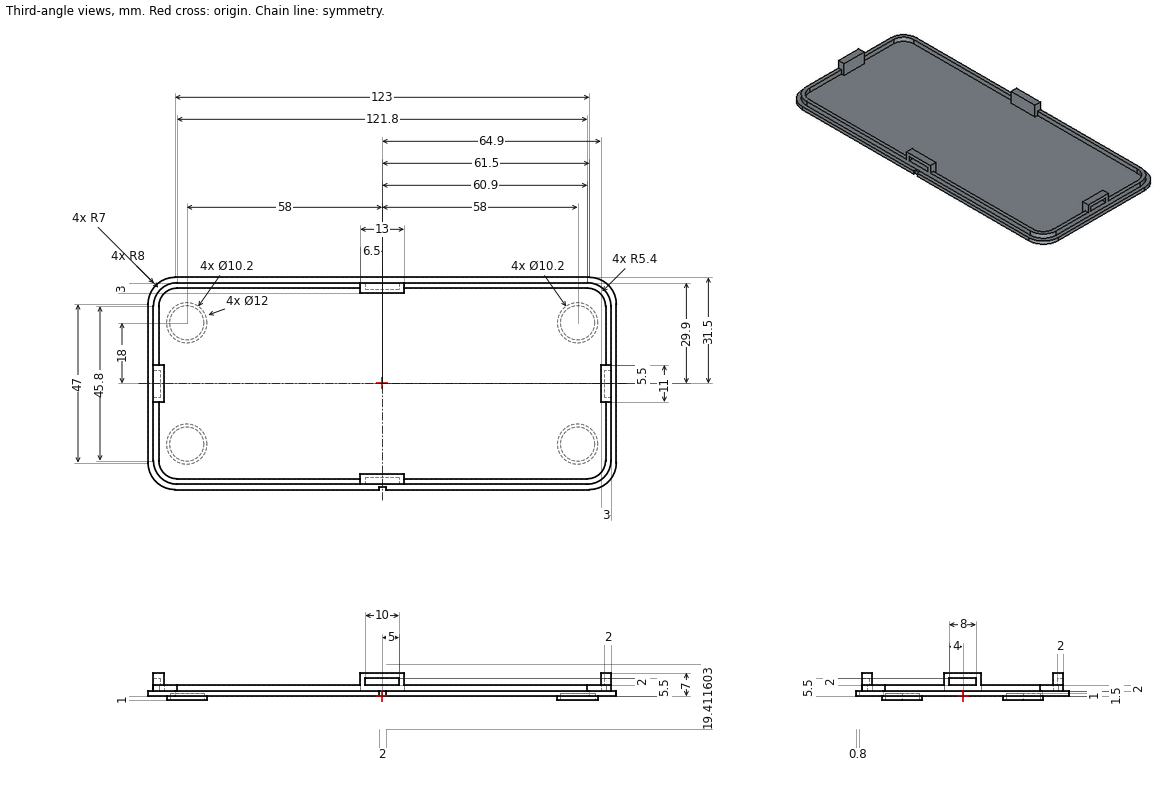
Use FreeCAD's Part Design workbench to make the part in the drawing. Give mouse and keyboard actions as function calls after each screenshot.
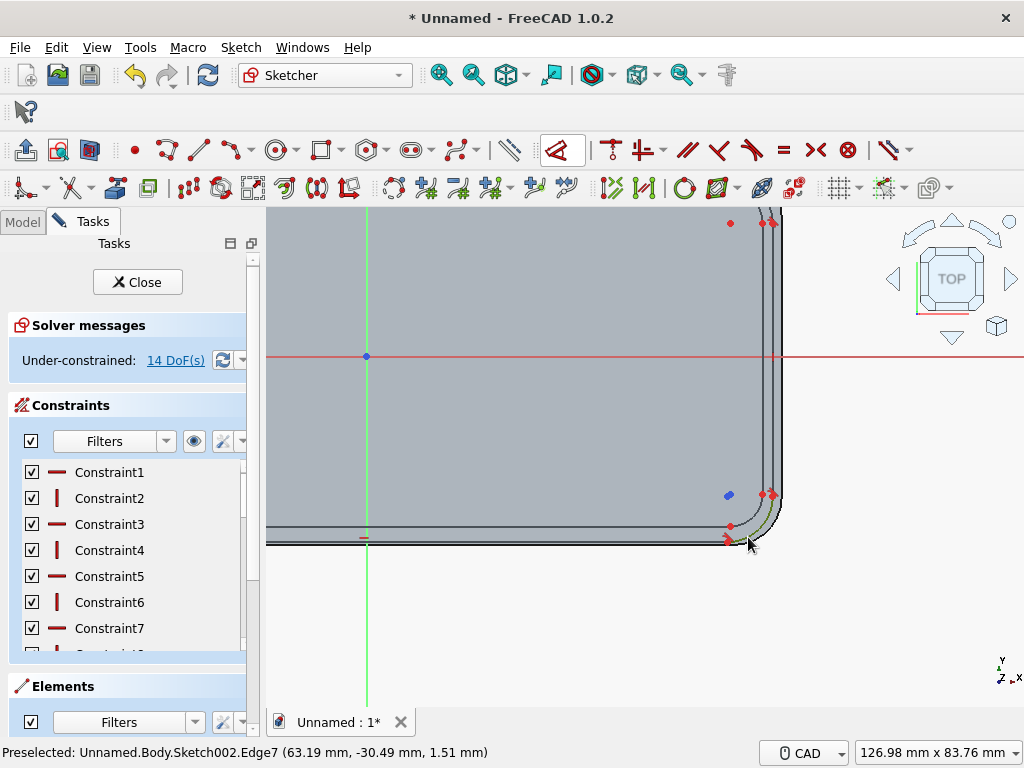
click(745, 523)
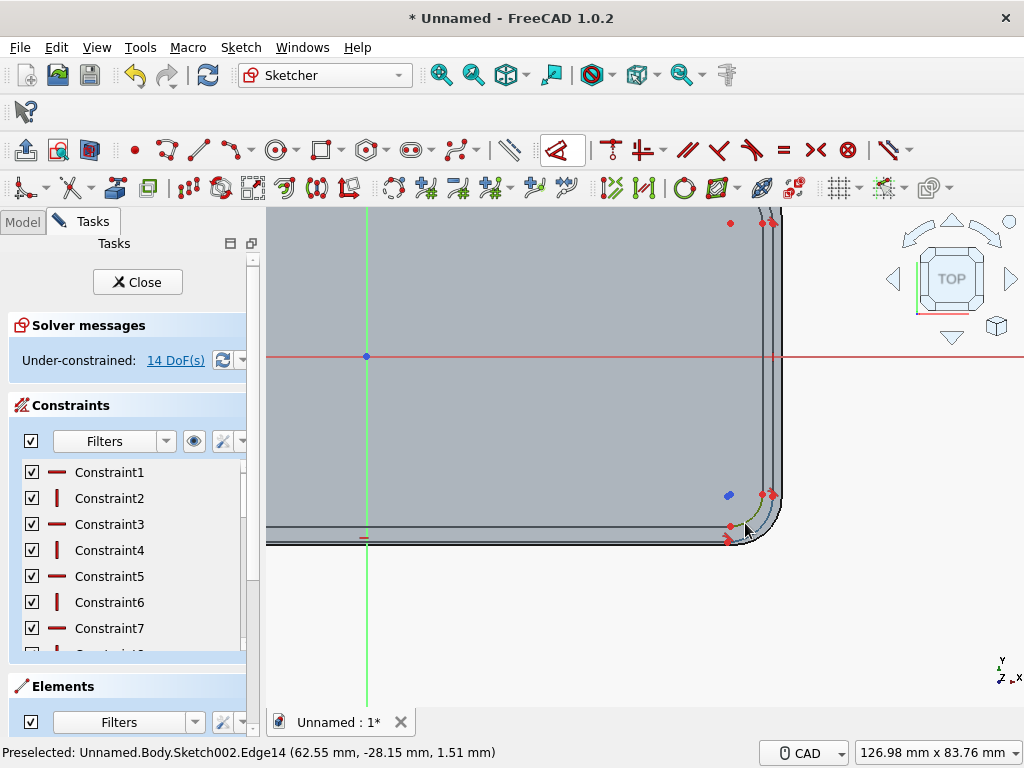
click(612, 150)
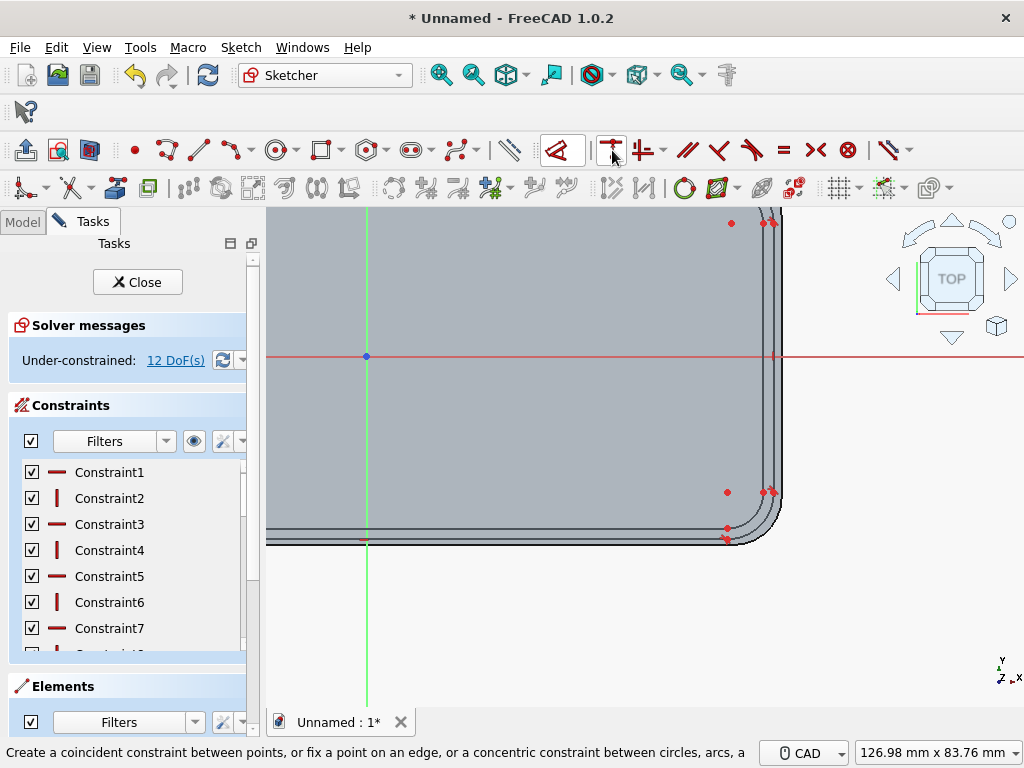
scroll(748, 539, down, 4)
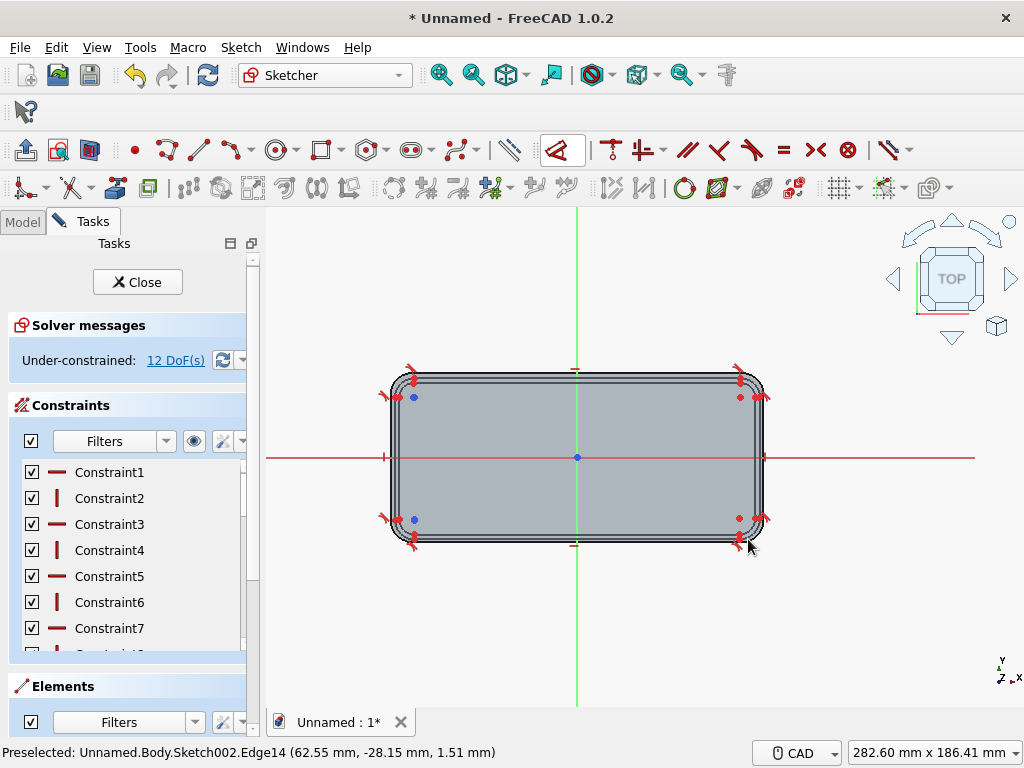
scroll(397, 529, up, 6)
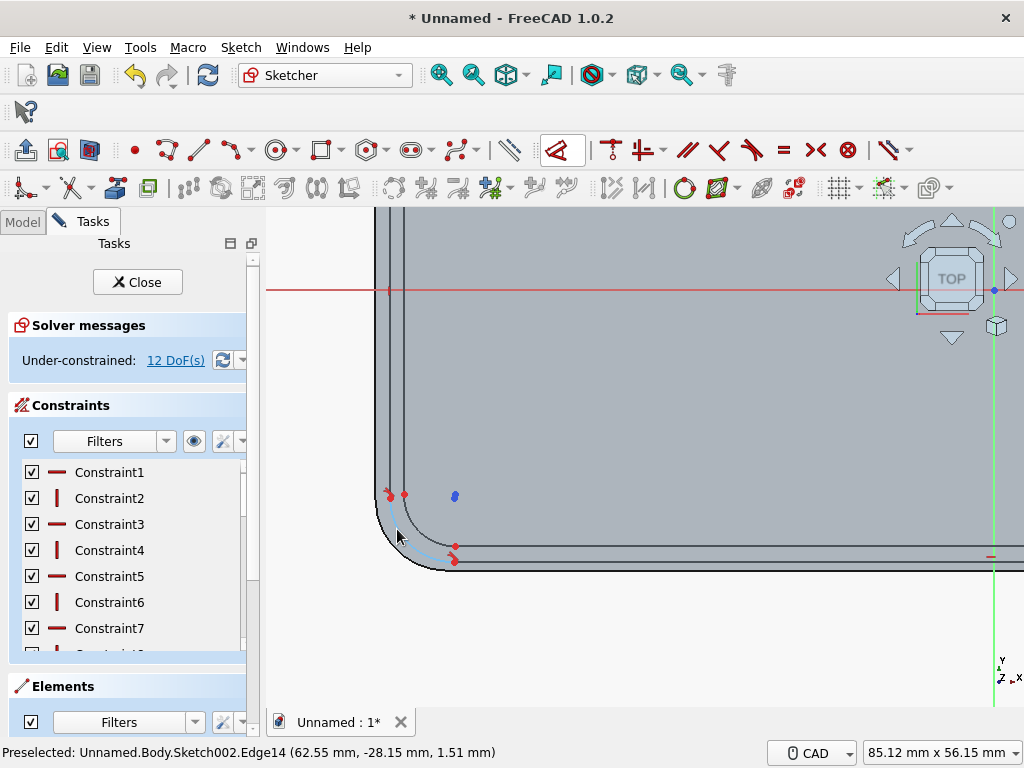
click(397, 527)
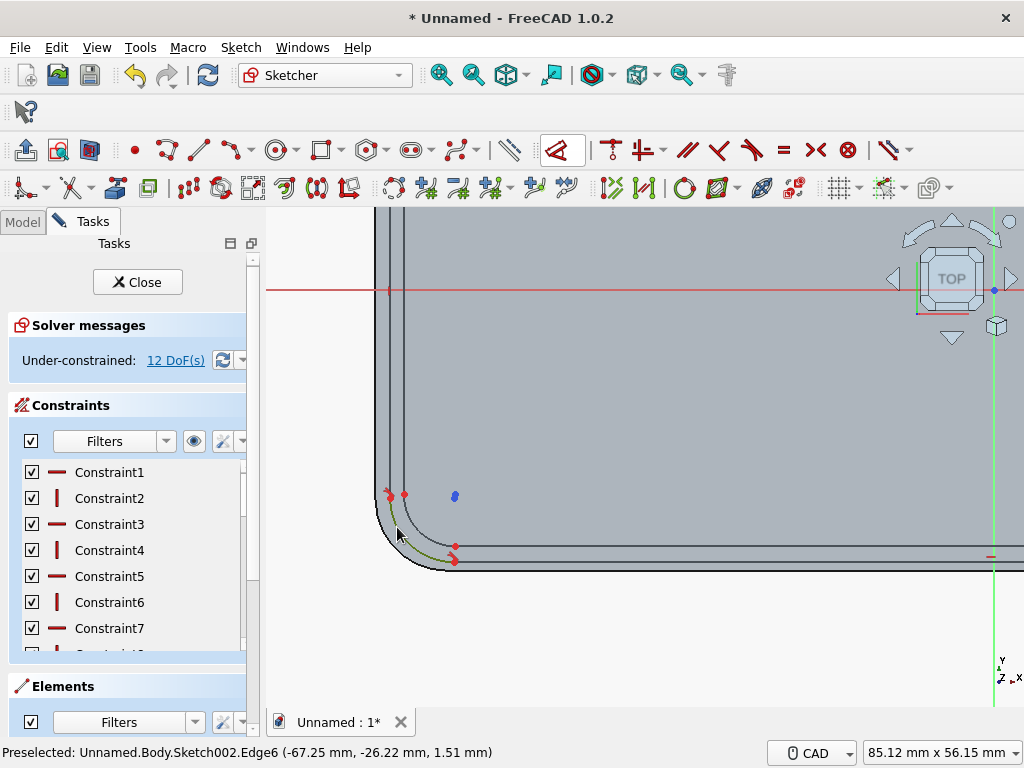
click(410, 518)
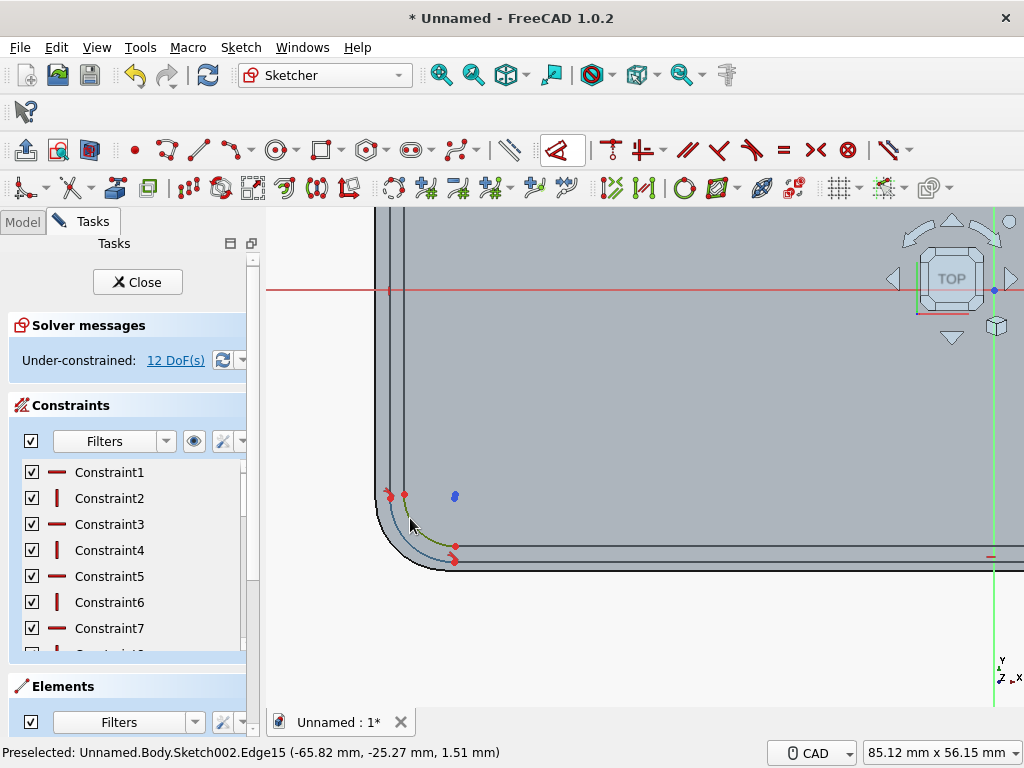
key(c)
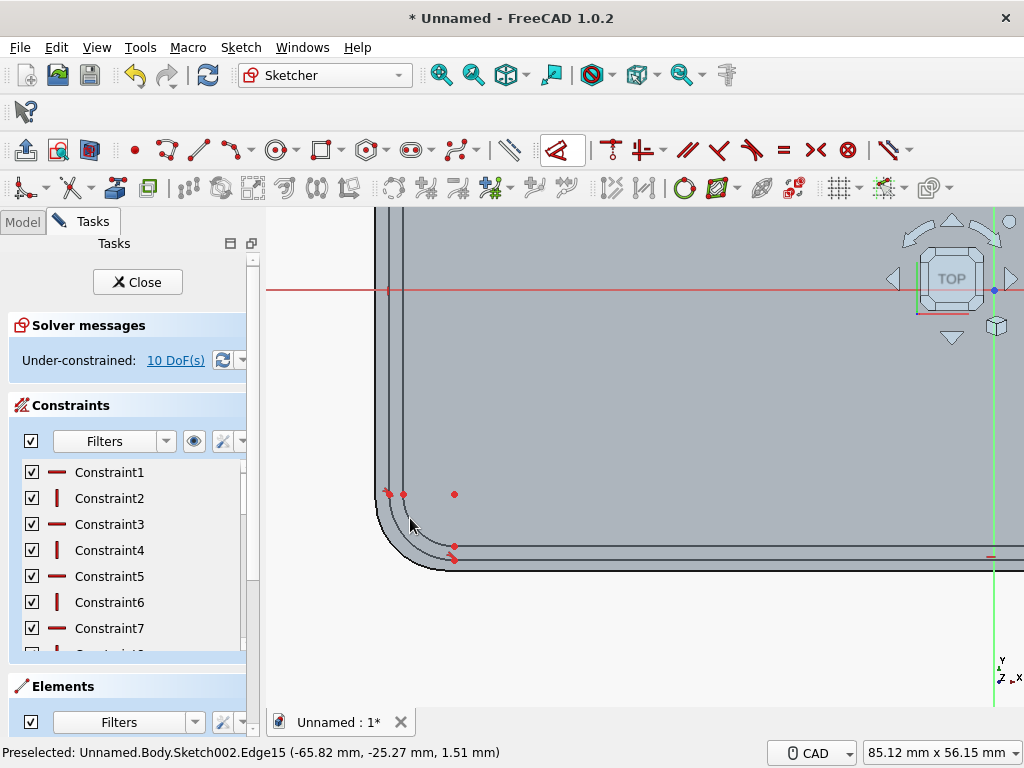
scroll(396, 529, down, 6)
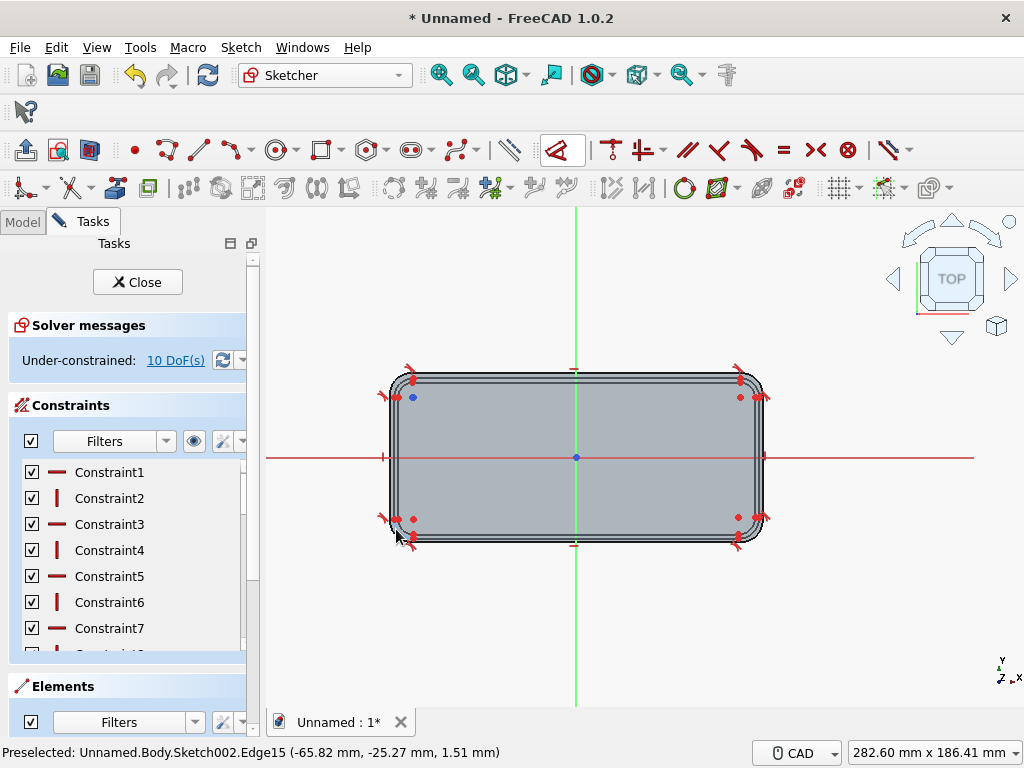
scroll(405, 380, up, 7)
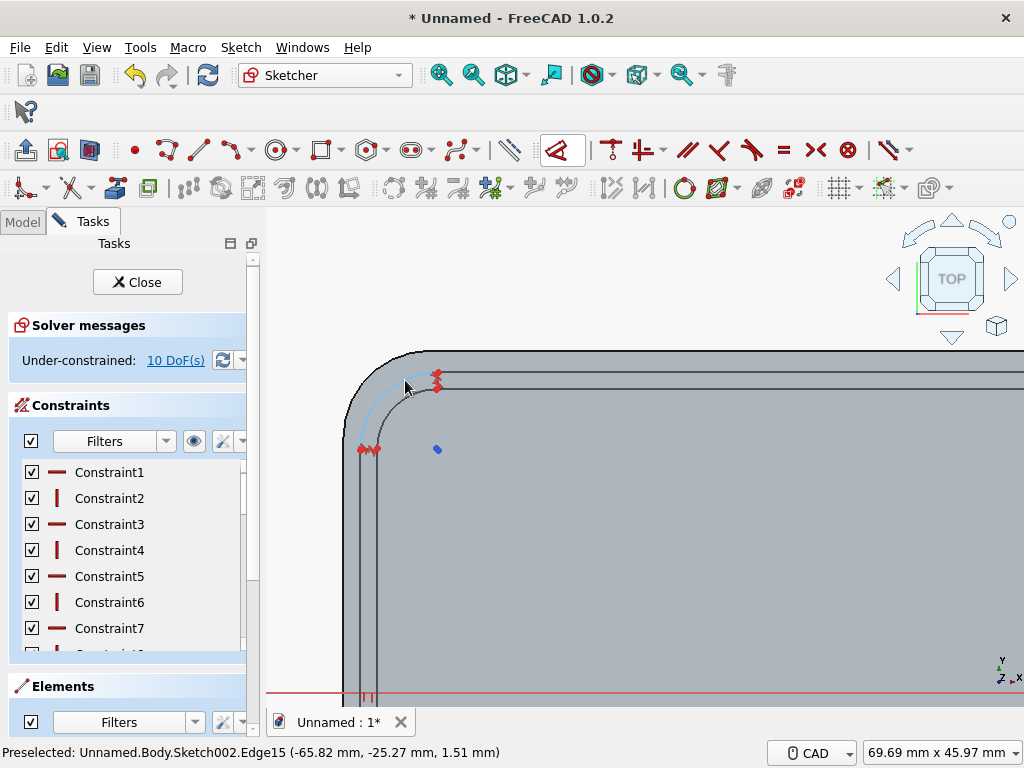
click(403, 381)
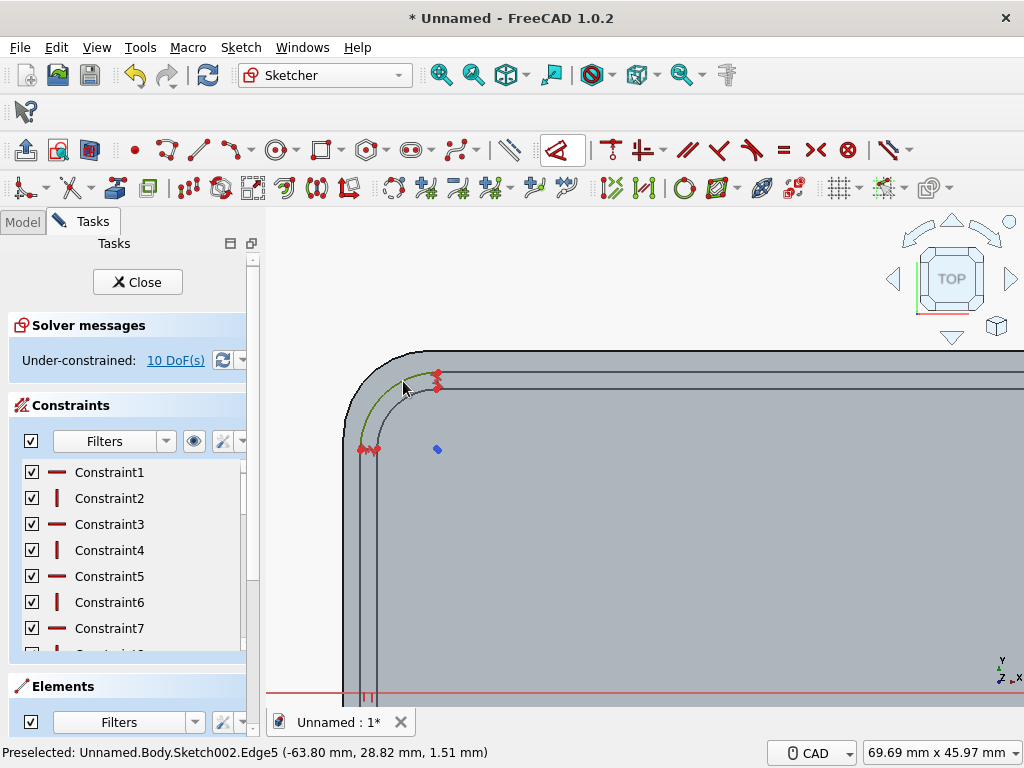
scroll(405, 380, down, 7)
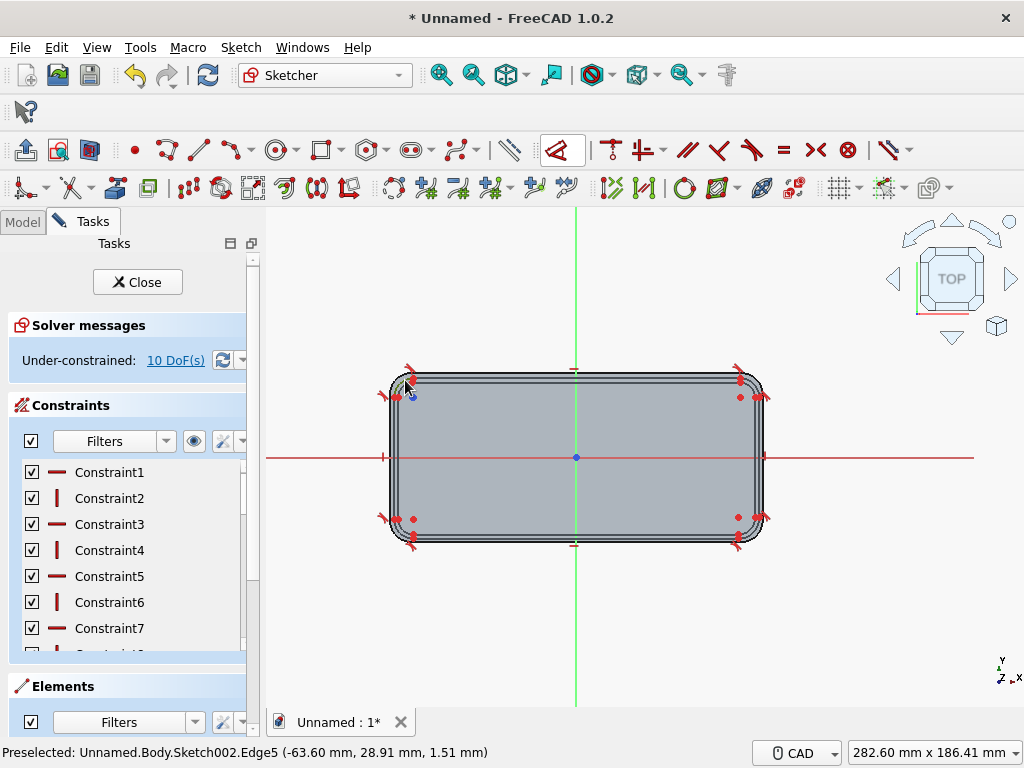
scroll(396, 528, up, 6)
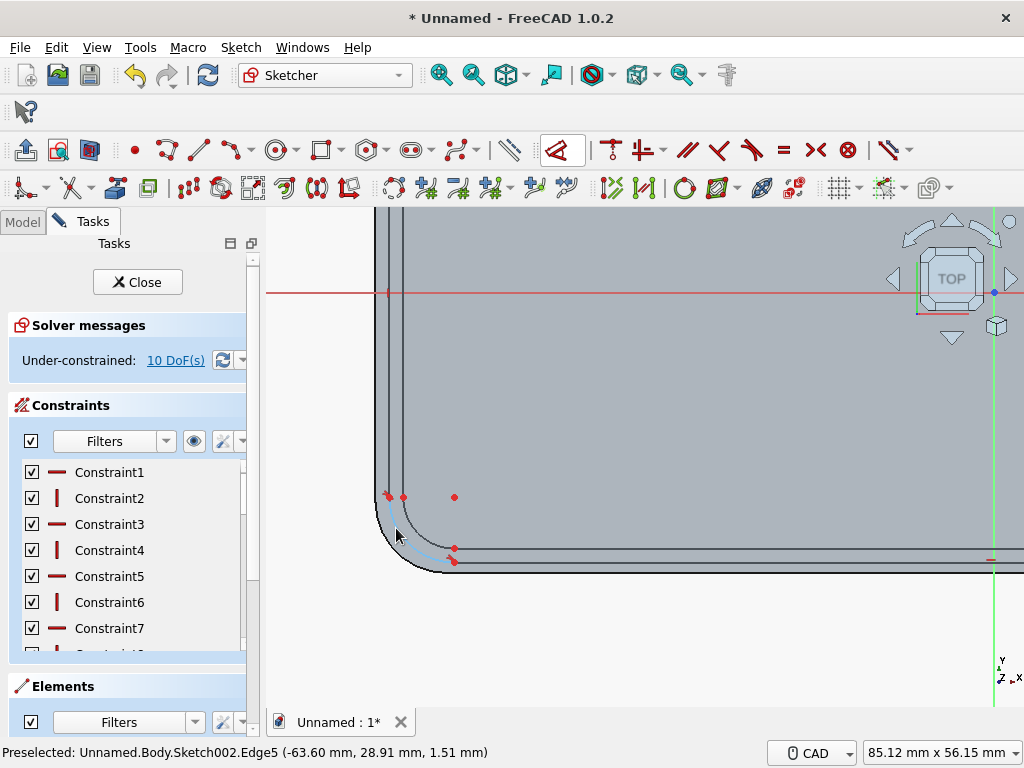
click(396, 527)